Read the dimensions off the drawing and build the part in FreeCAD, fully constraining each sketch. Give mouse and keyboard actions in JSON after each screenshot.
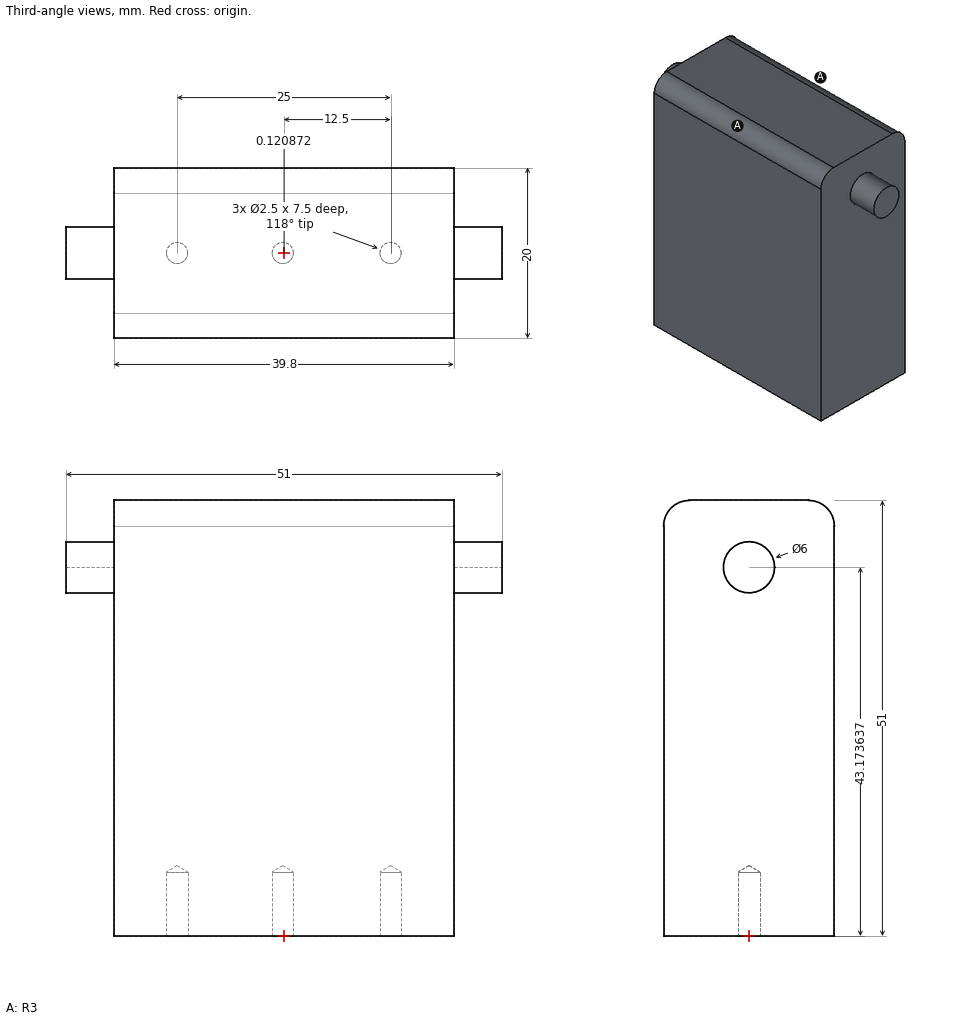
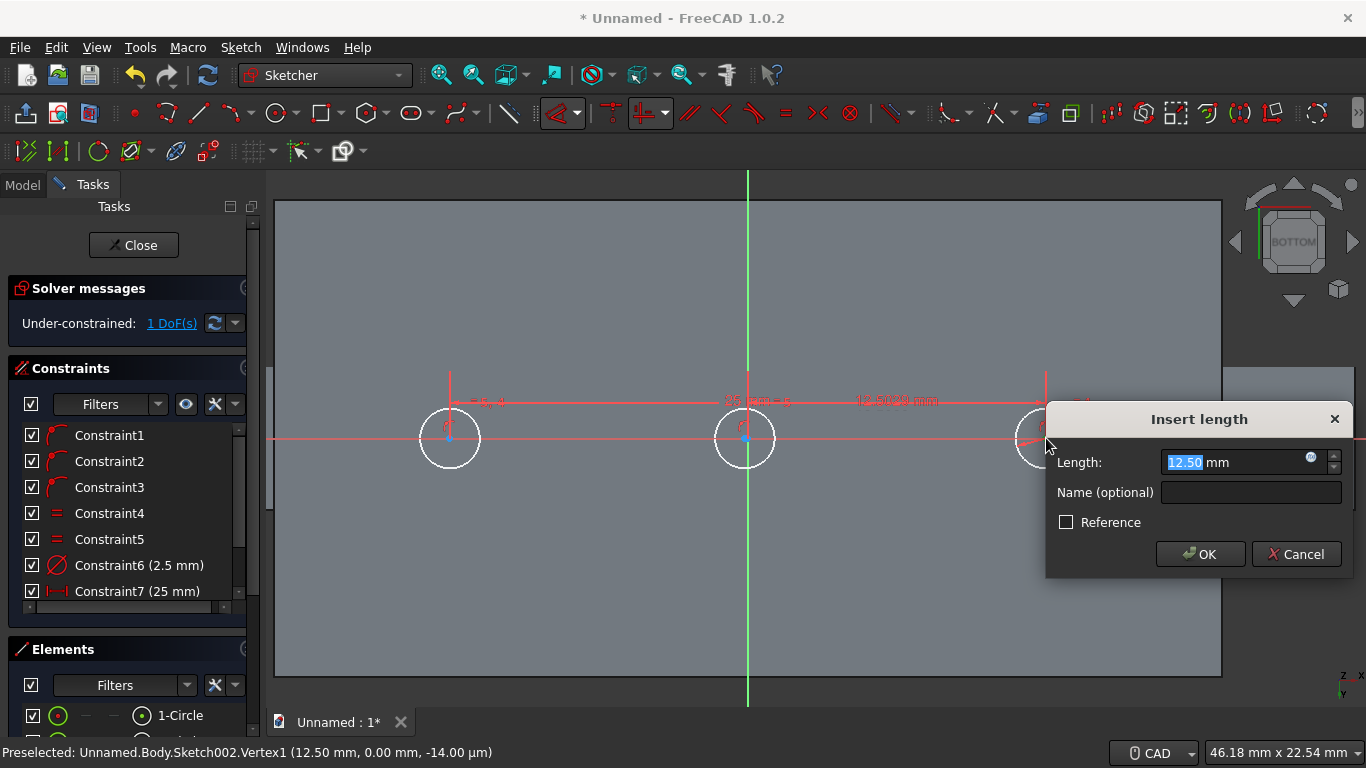
{"action": "type", "text": "12.5"}
{"action": "key", "text": "Return"}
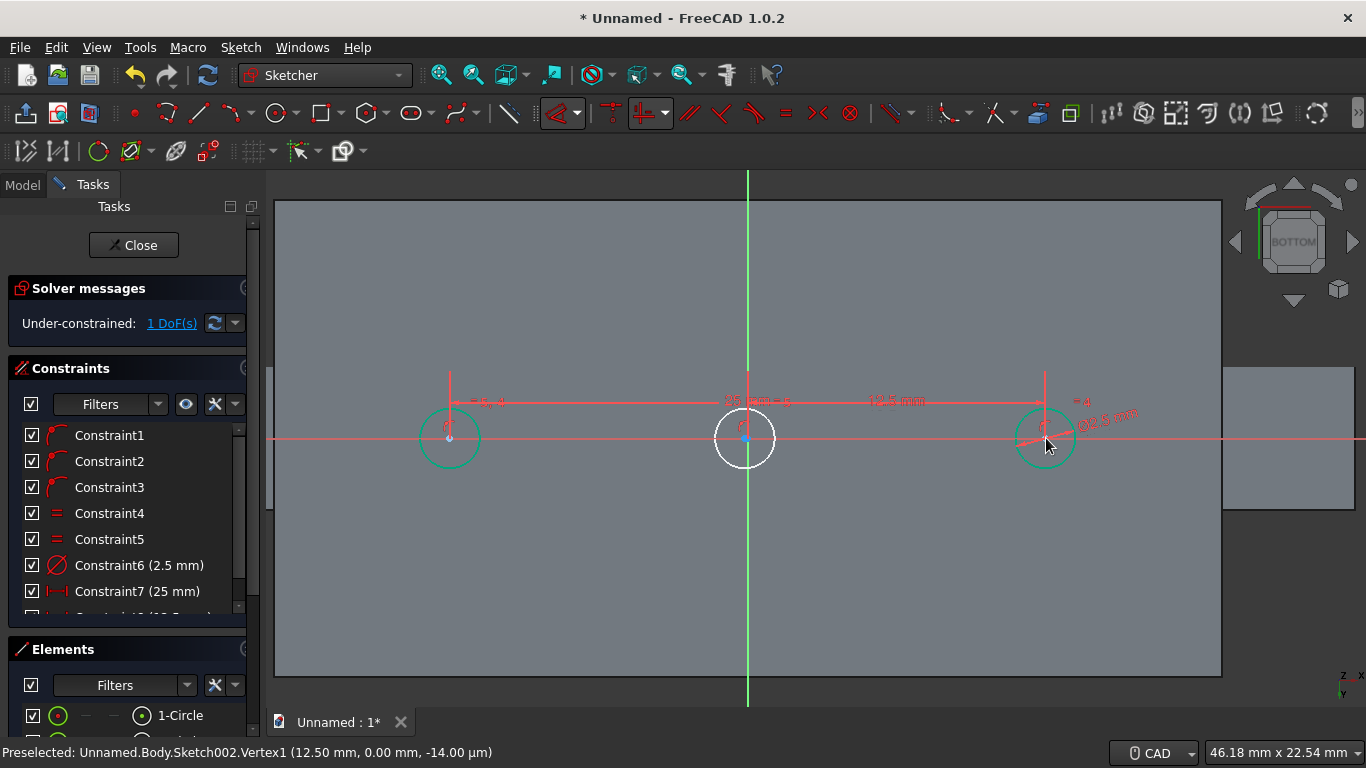
{"action": "scroll", "coordinate": [745, 438], "scroll_direction": "up", "scroll_amount": 14}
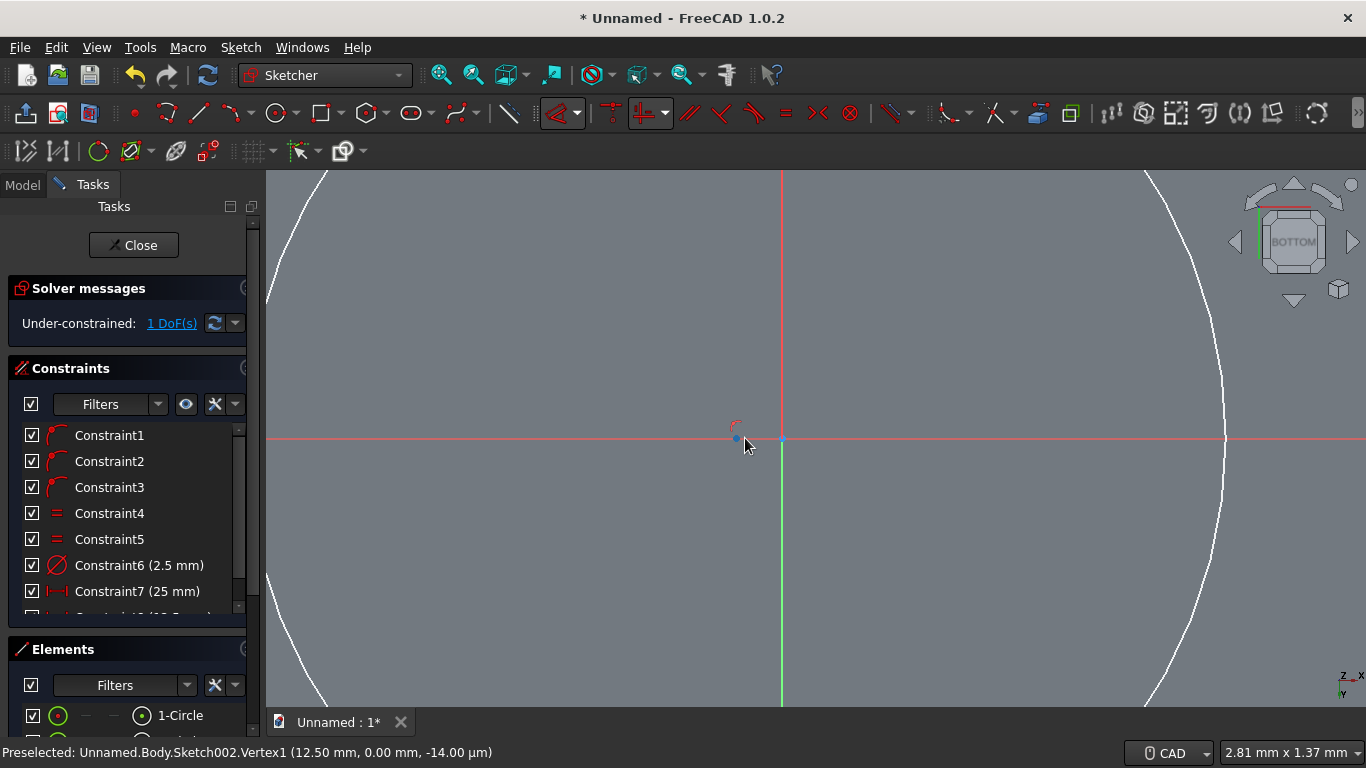
{"action": "left_click", "coordinate": [736, 438]}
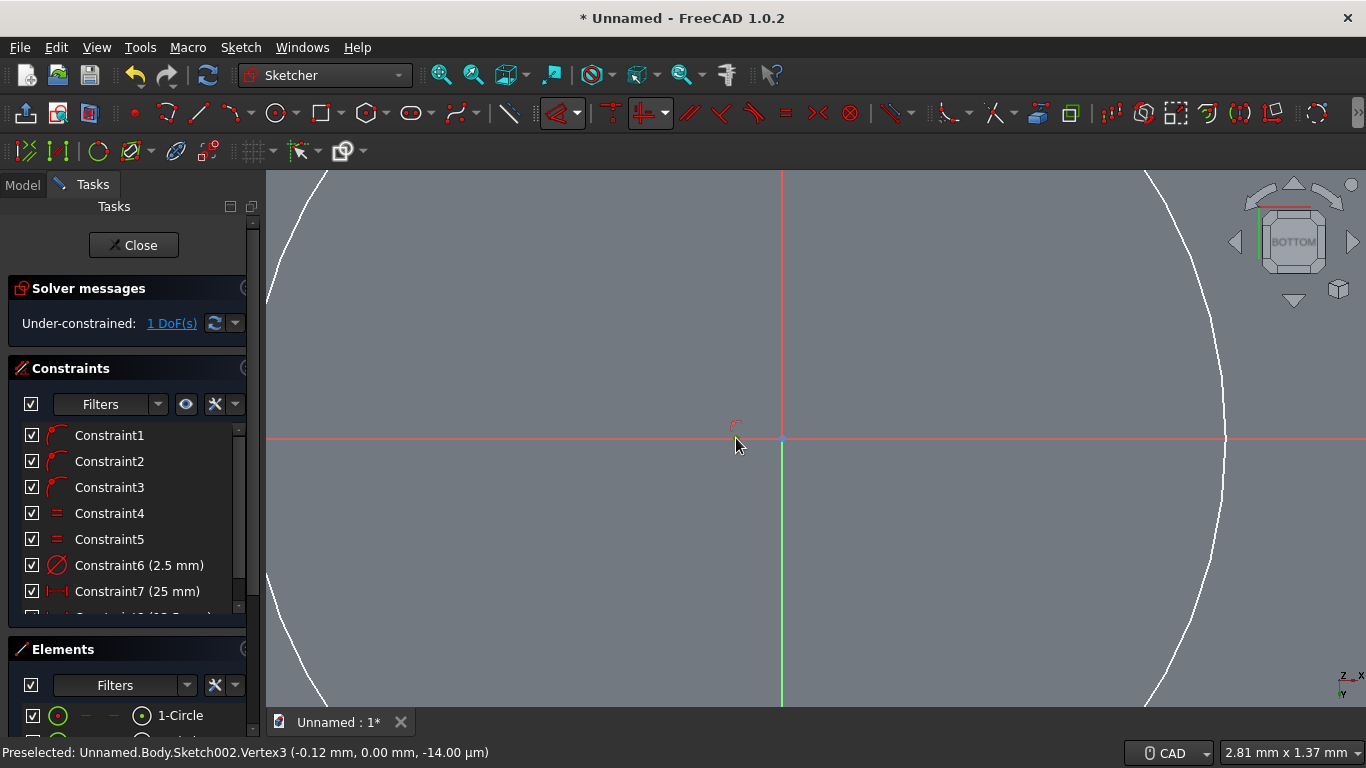
{"action": "key", "text": "l"}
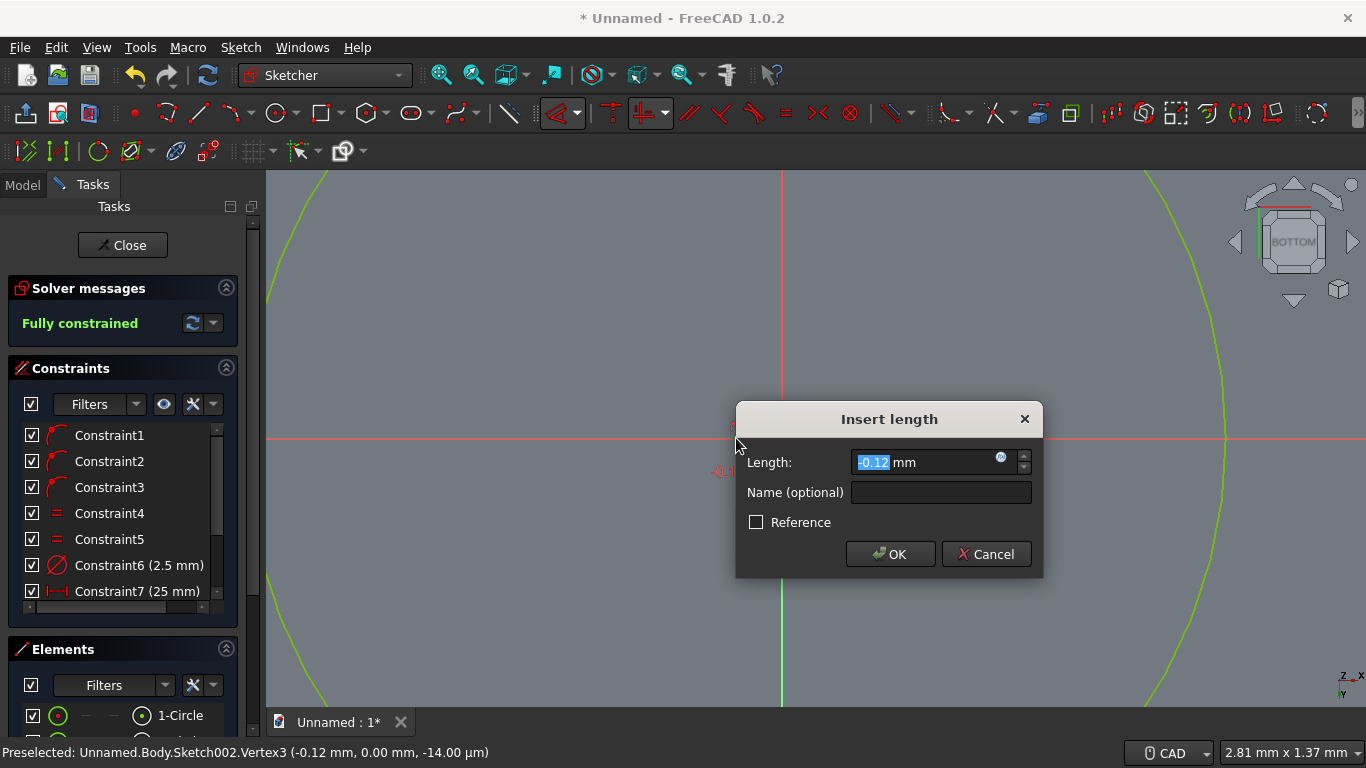
{"action": "type", "text": "-0.120872"}
{"action": "key", "text": "Return"}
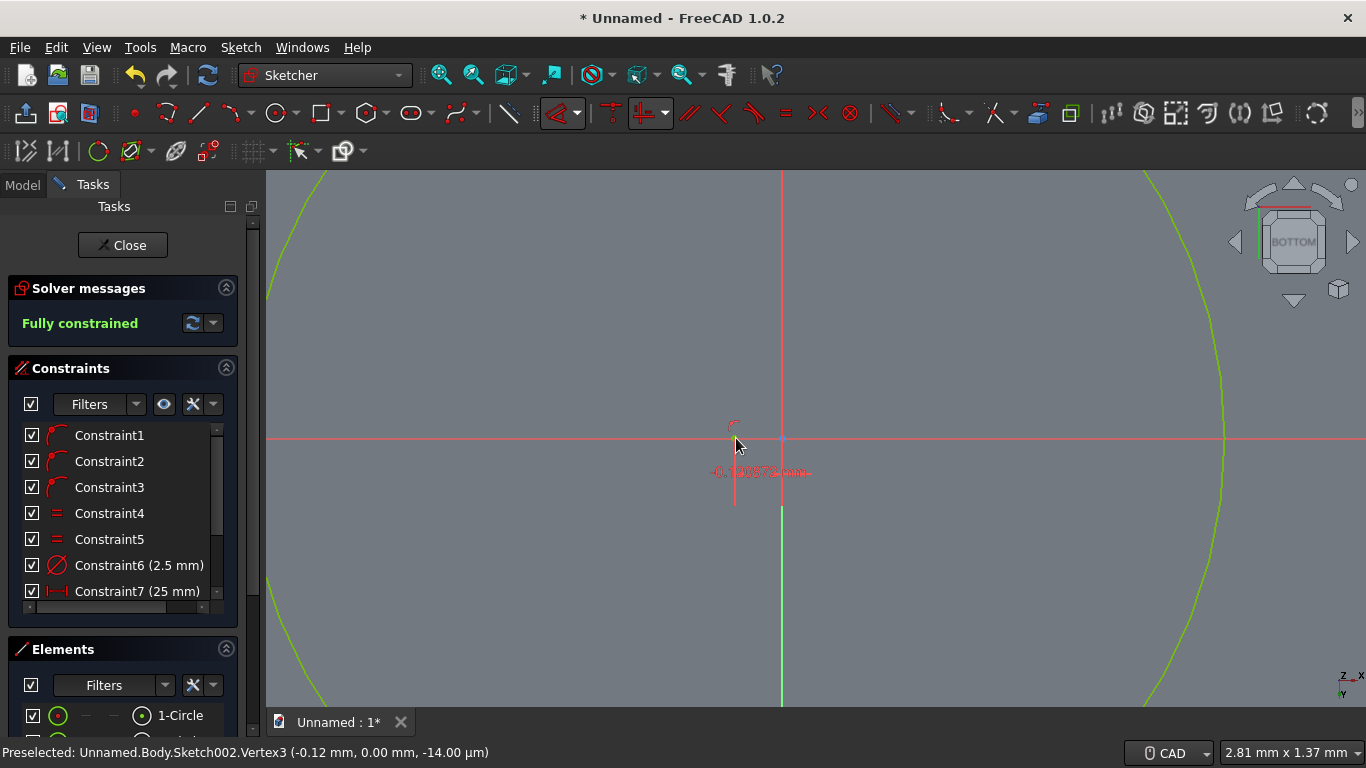
{"action": "left_click", "coordinate": [123, 245]}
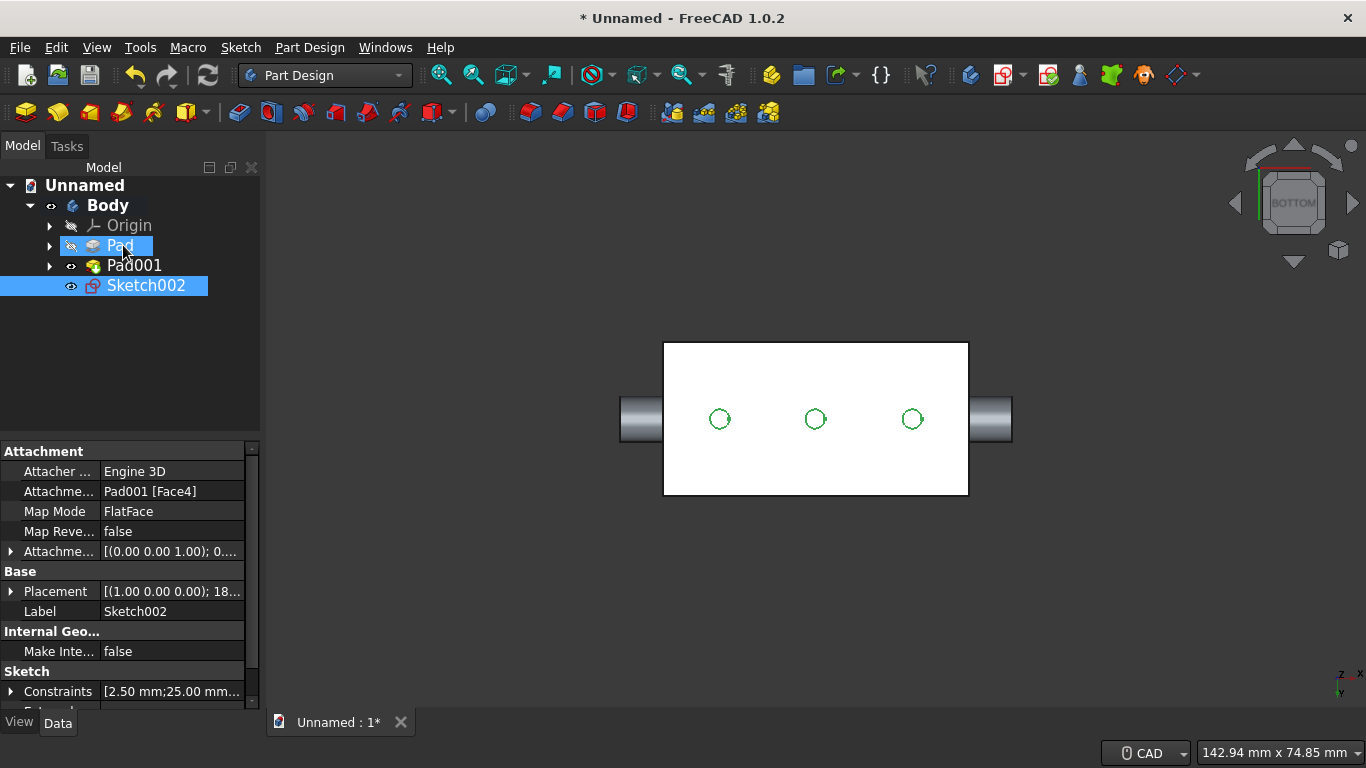
{"action": "left_click", "coordinate": [272, 112]}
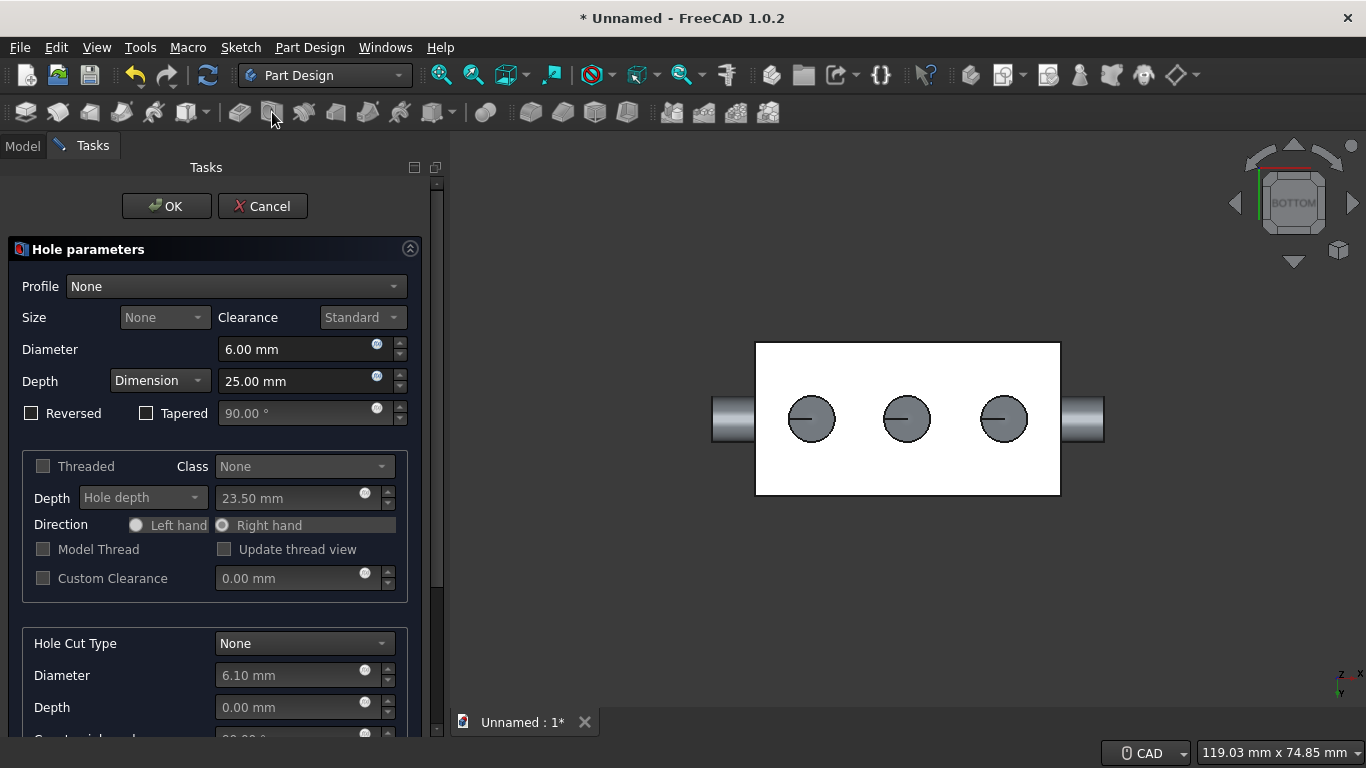
{"action": "triple_click", "coordinate": [305, 349]}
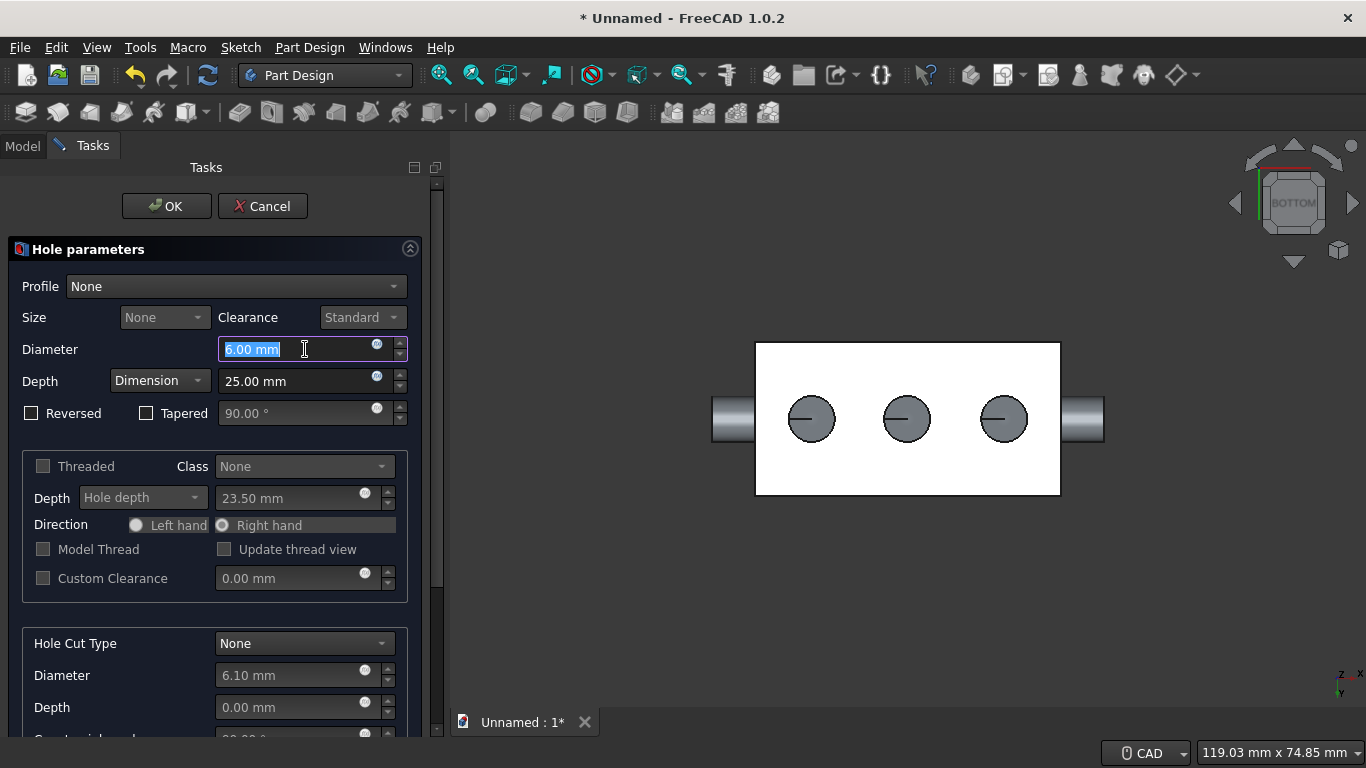
{"action": "type", "text": "2.5"}
{"action": "key", "text": "Tab"}